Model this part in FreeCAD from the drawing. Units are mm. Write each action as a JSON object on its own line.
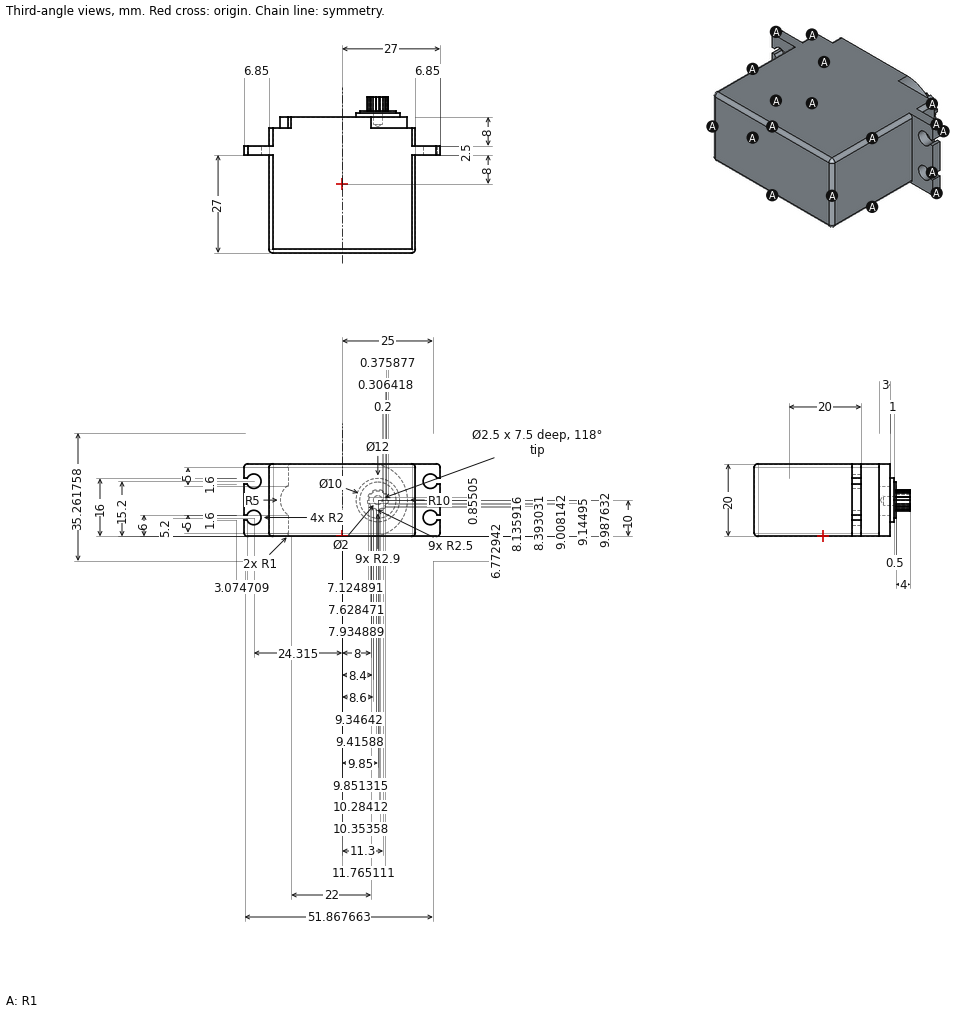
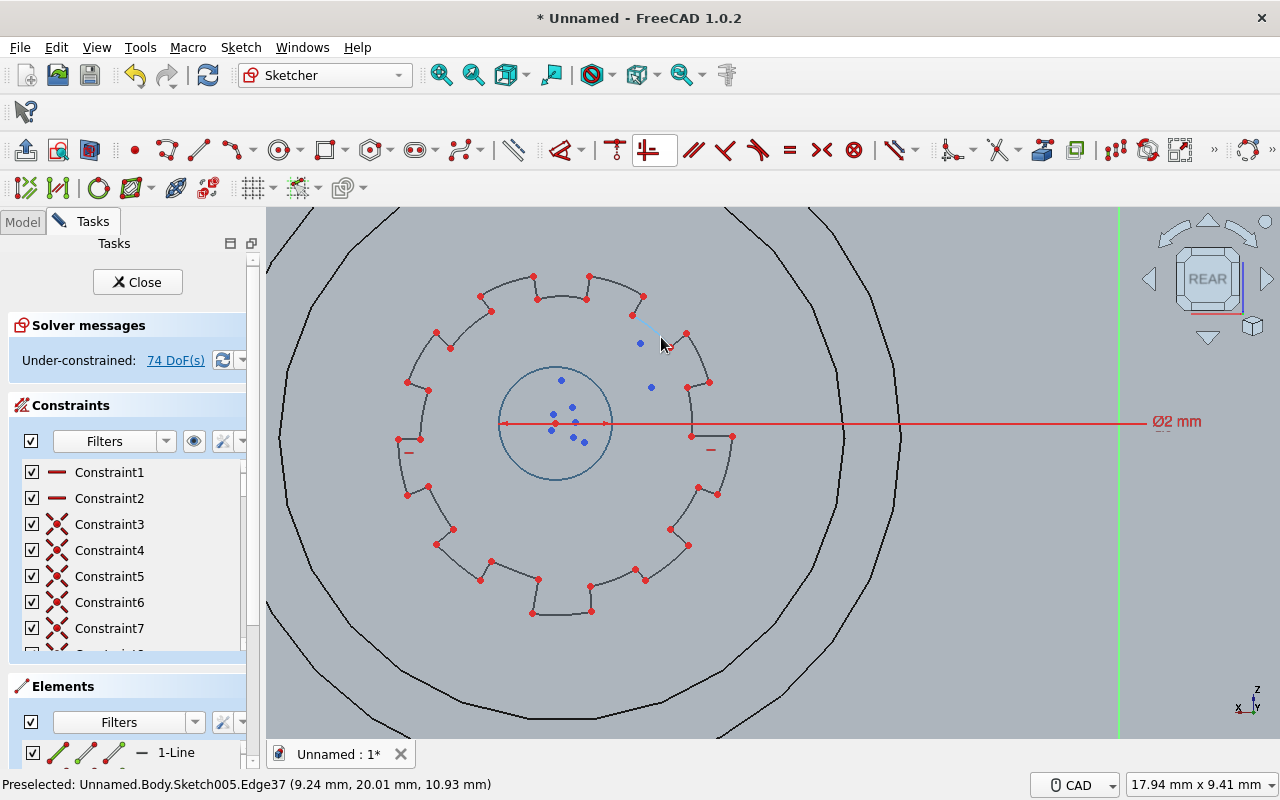
{"action": "left_click", "coordinate": [661, 336]}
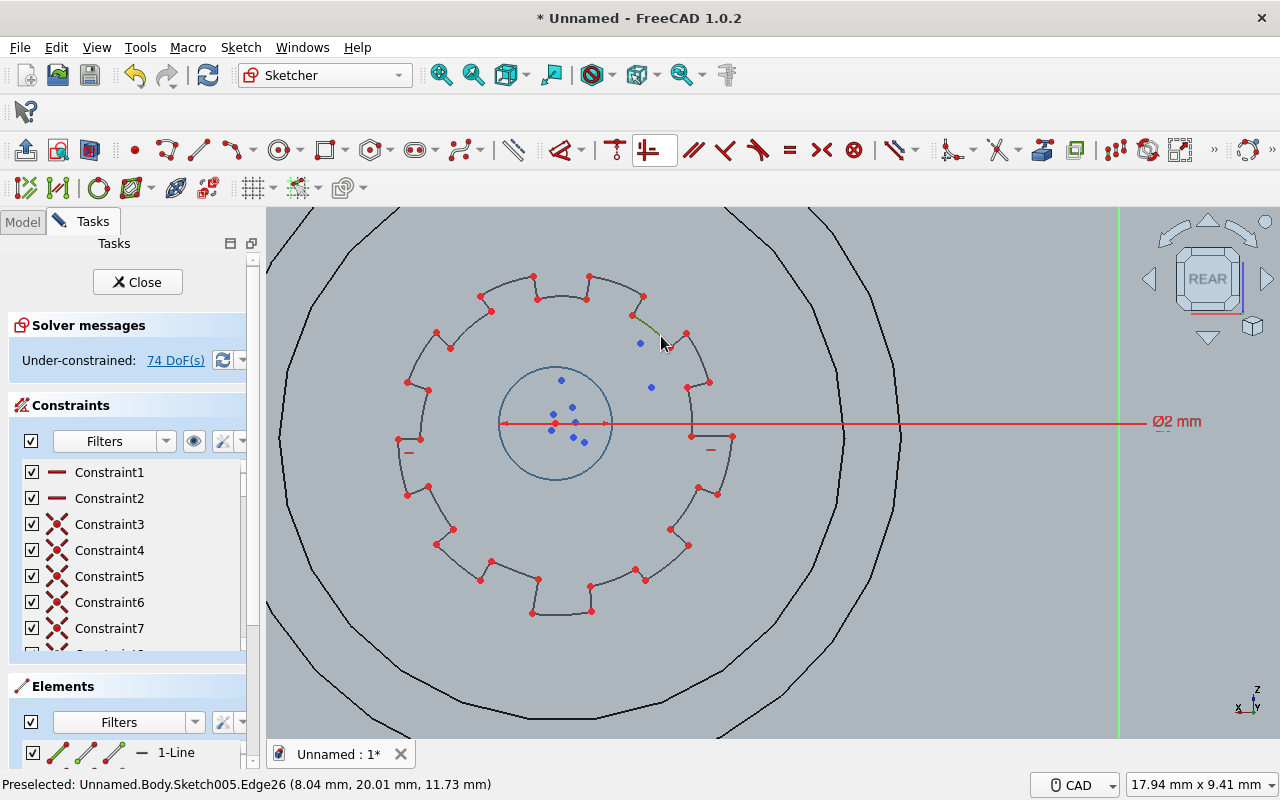
{"action": "left_click", "coordinate": [616, 150]}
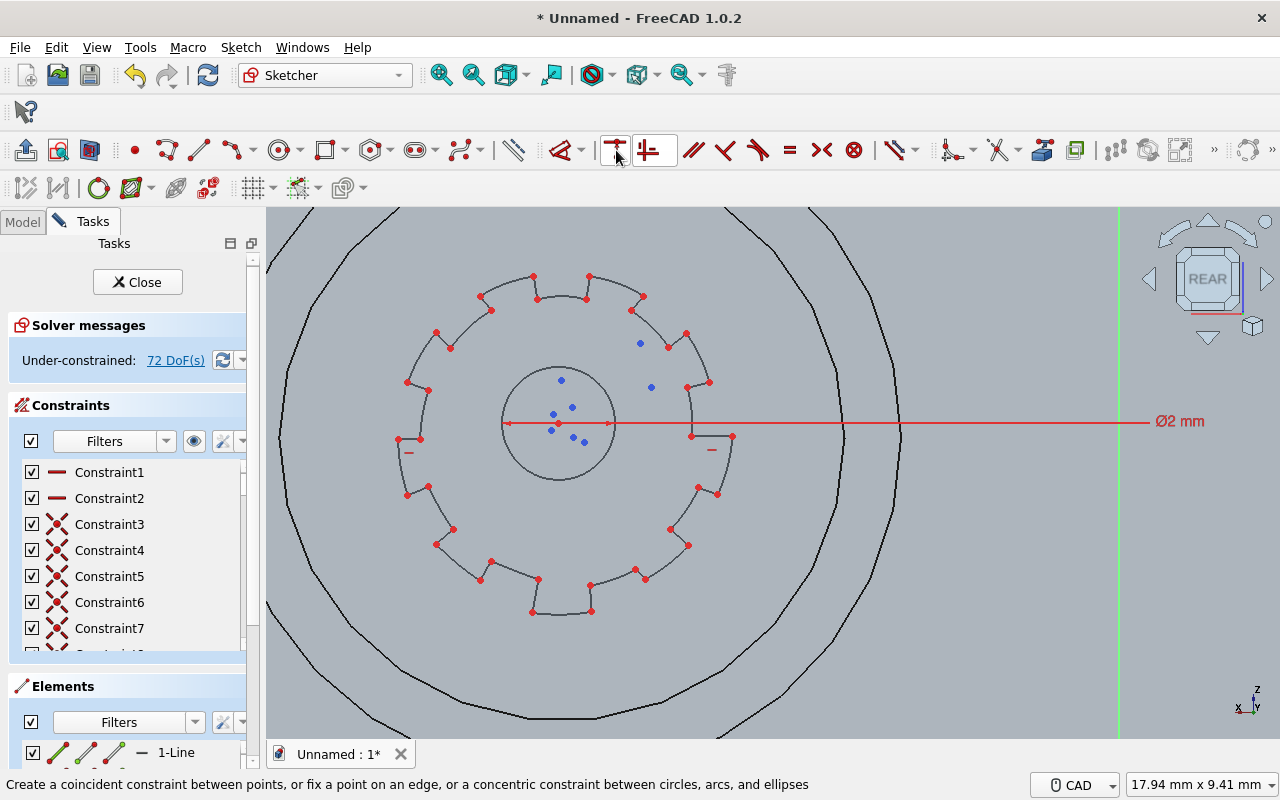
{"action": "left_click", "coordinate": [598, 383]}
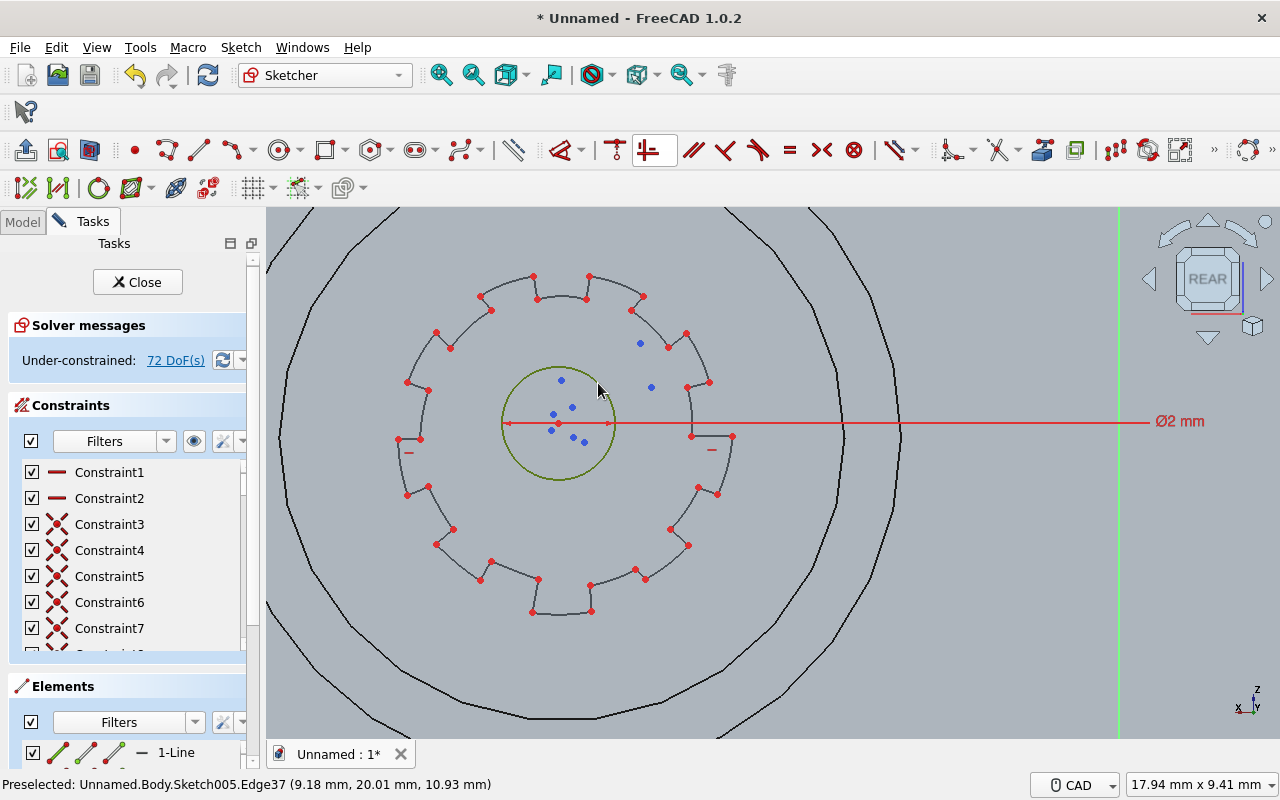
{"action": "left_click", "coordinate": [629, 288]}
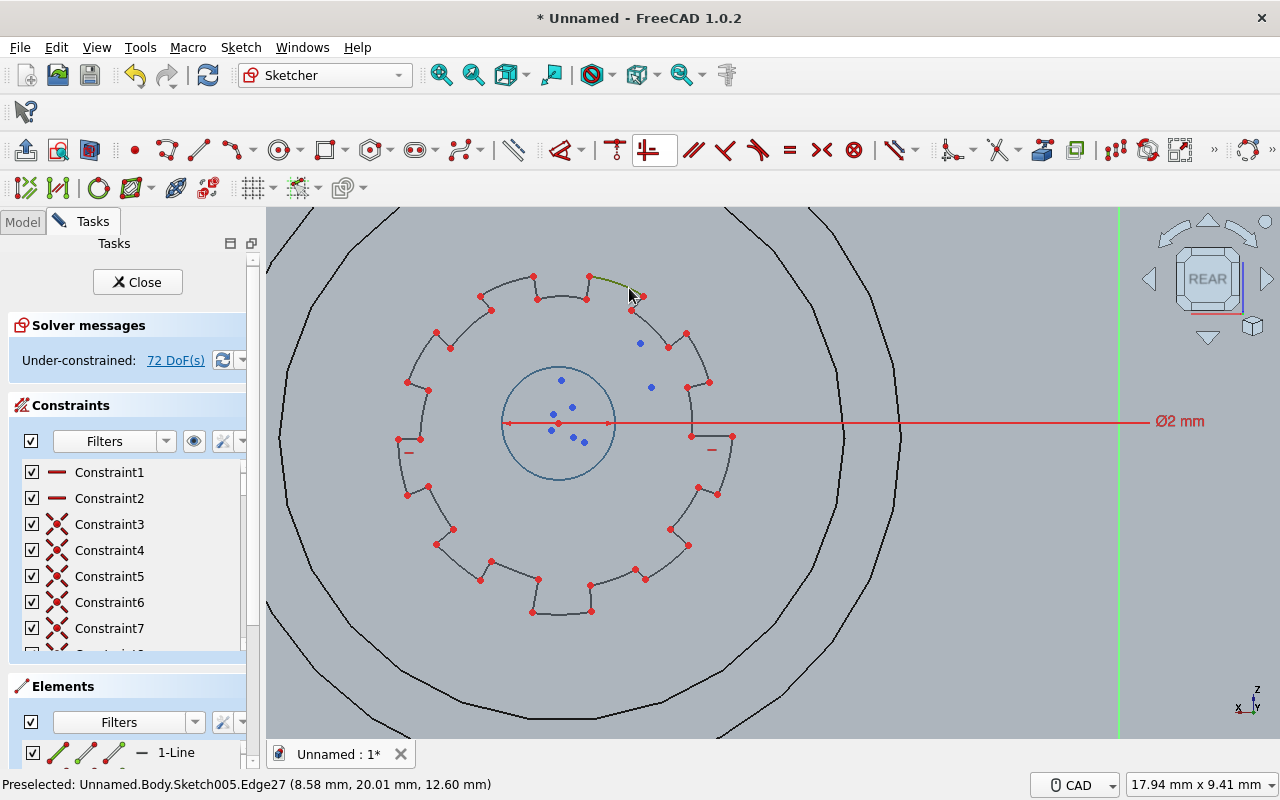
{"action": "left_click", "coordinate": [616, 150]}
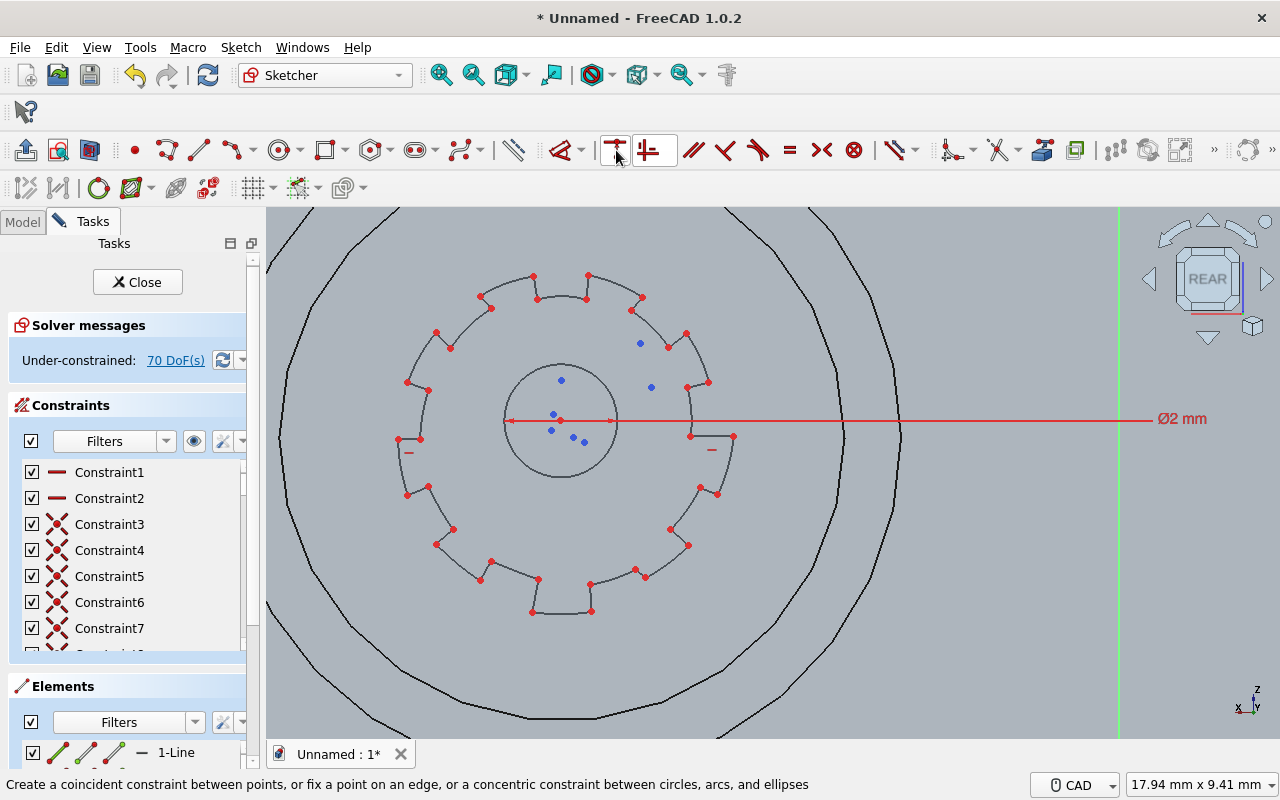
{"action": "left_click", "coordinate": [601, 381]}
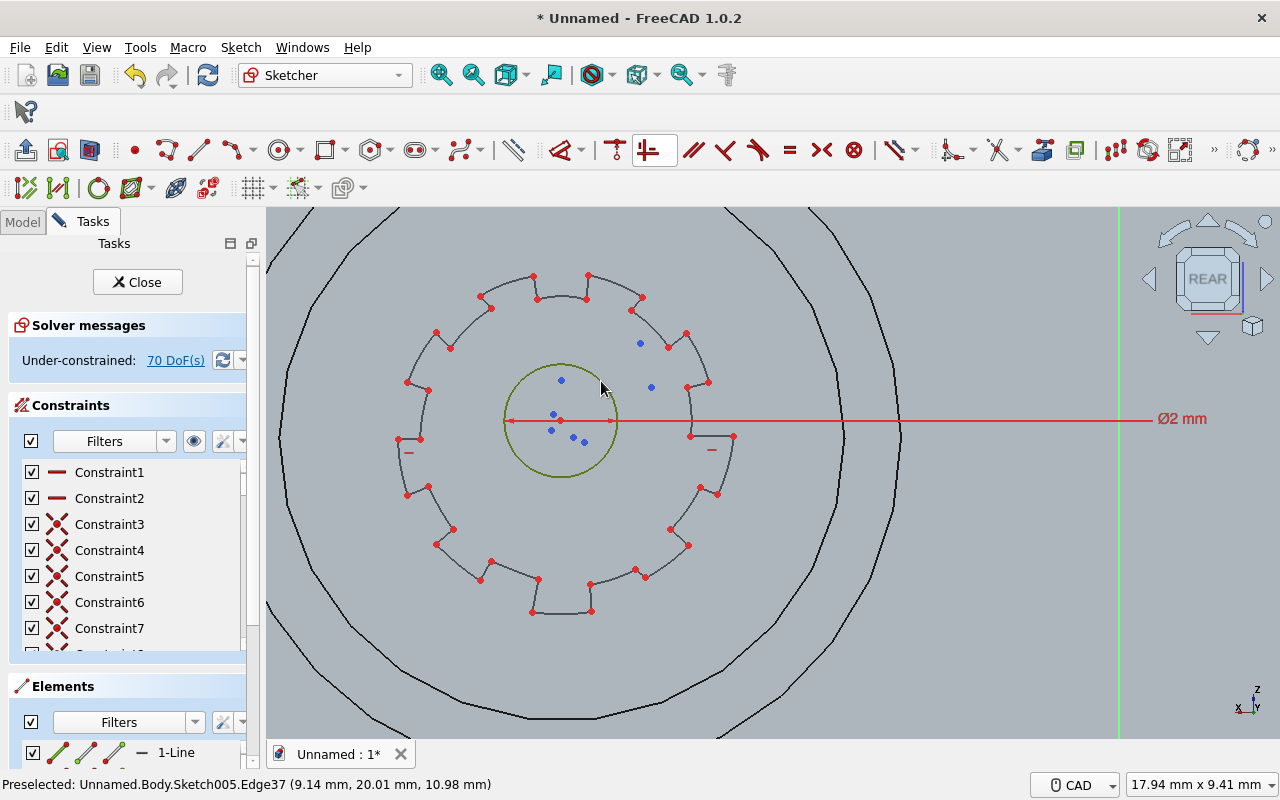
{"action": "left_click", "coordinate": [572, 297]}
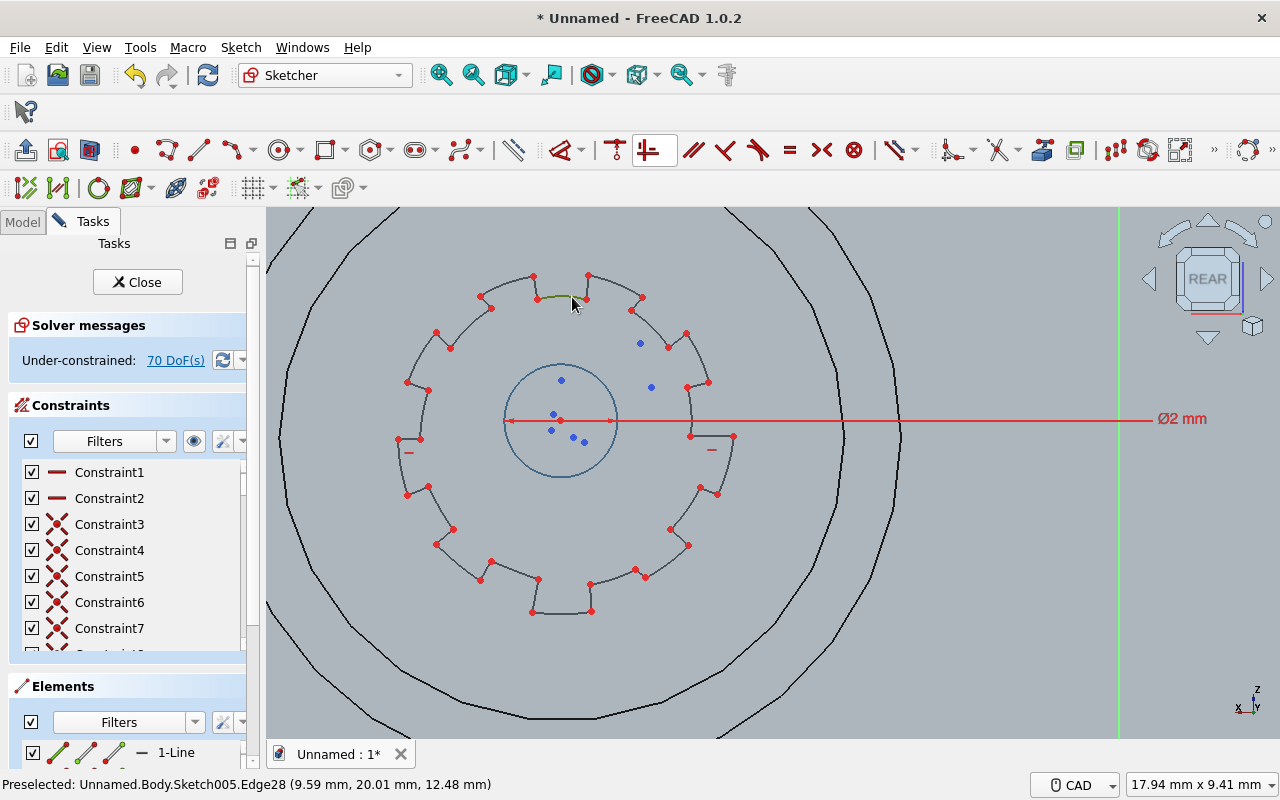
{"action": "left_click", "coordinate": [616, 150]}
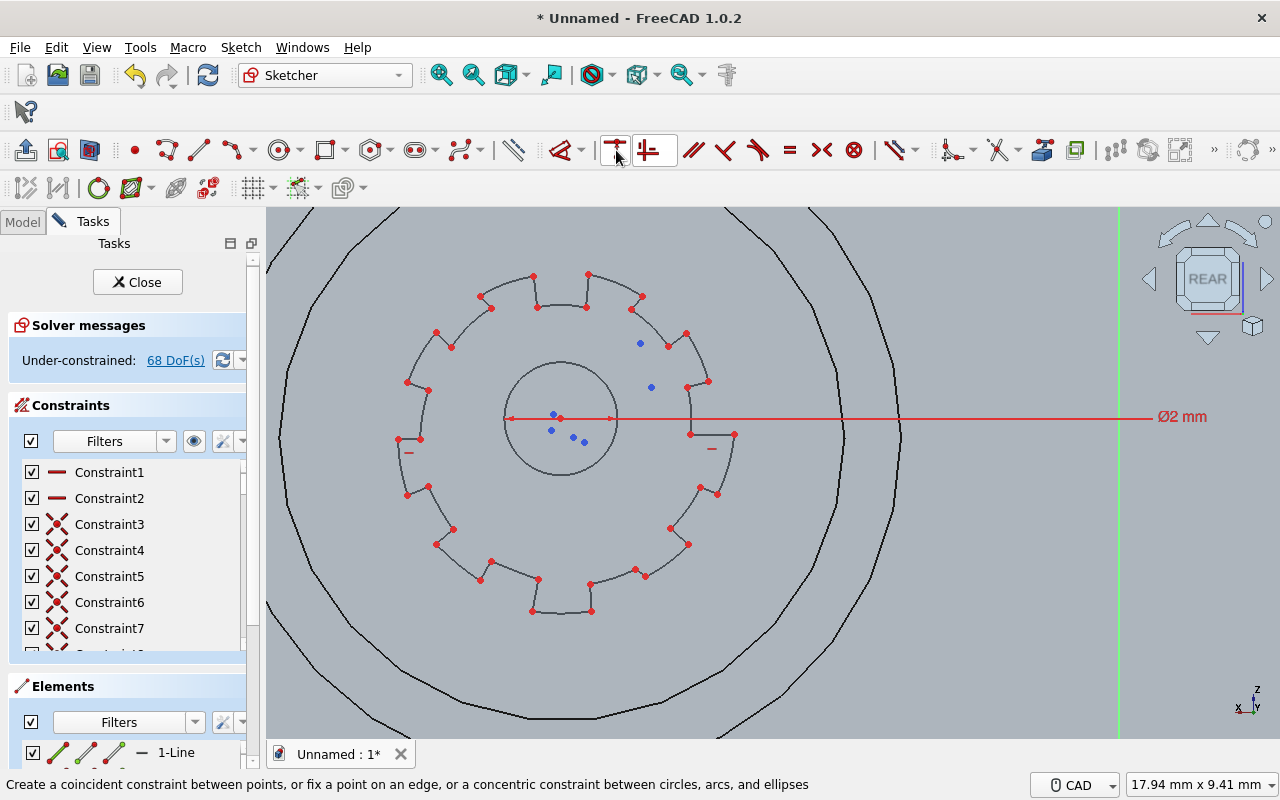
{"action": "left_click", "coordinate": [601, 379]}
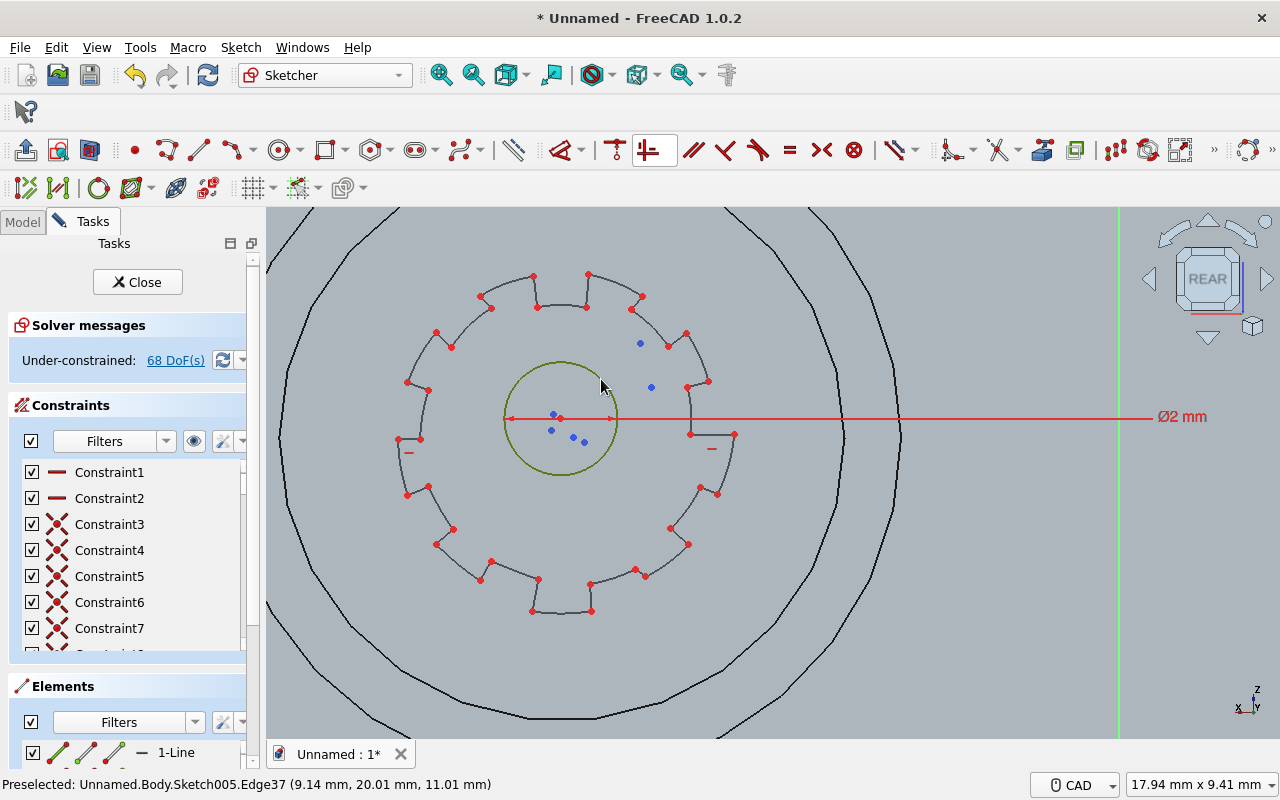
{"action": "left_click", "coordinate": [517, 280]}